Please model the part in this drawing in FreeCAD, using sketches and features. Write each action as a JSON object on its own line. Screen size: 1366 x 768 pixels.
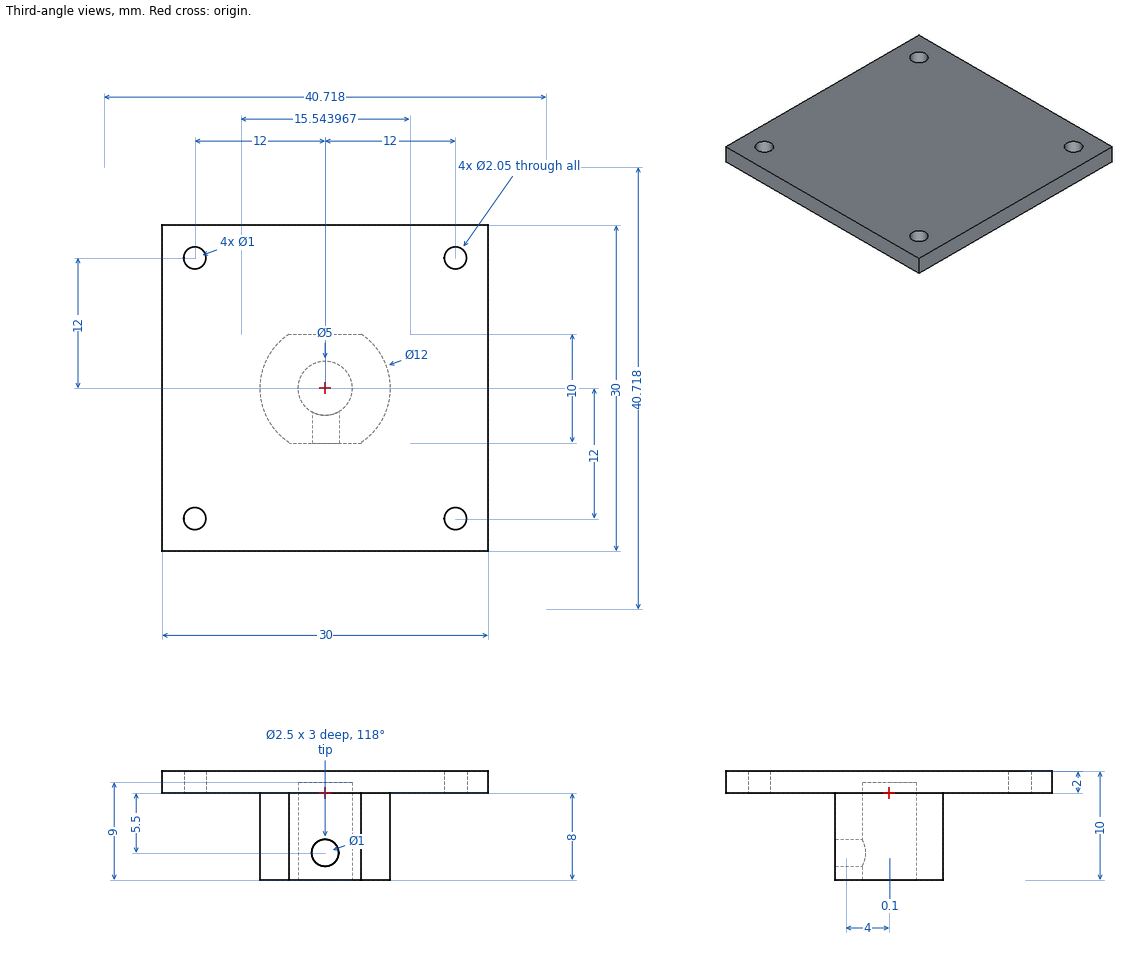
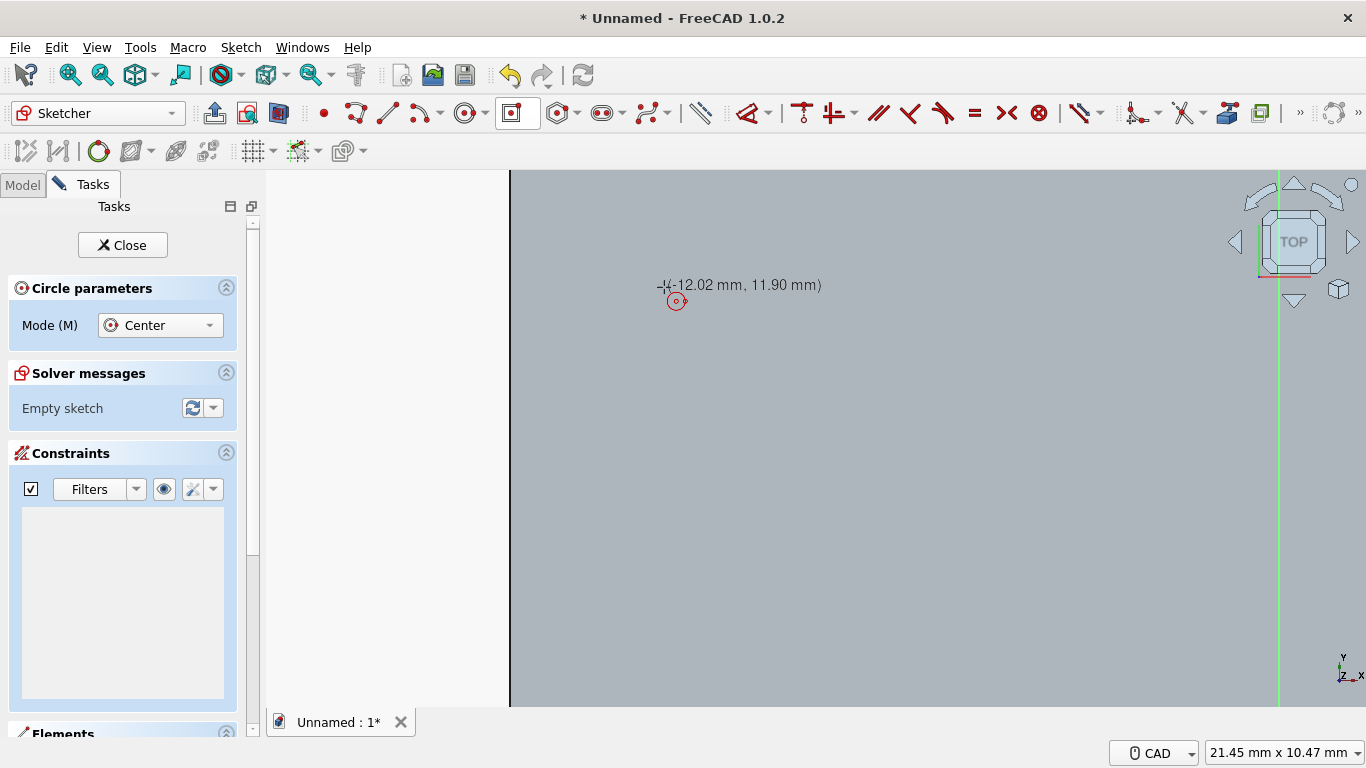
{"action": "scroll", "coordinate": [573, 287], "scroll_direction": "down", "scroll_amount": 7}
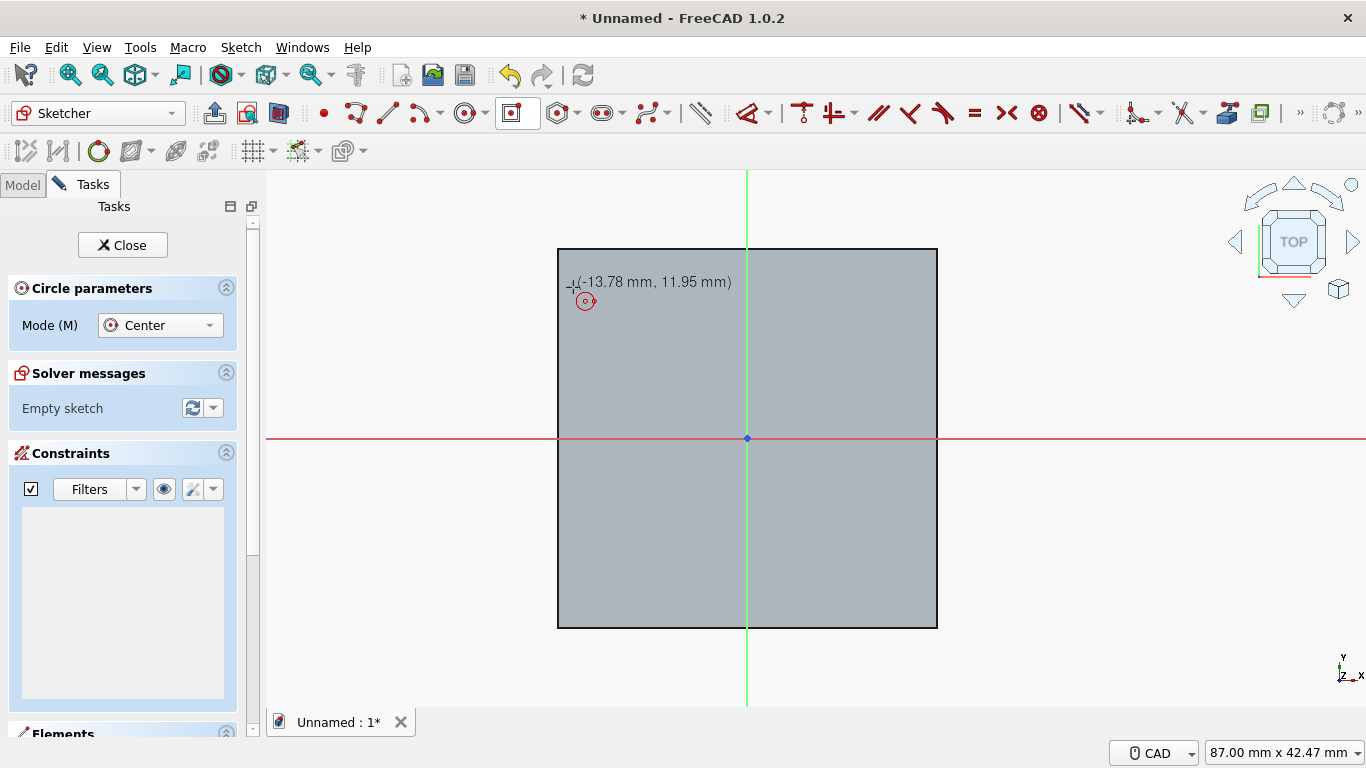
{"action": "left_click", "coordinate": [596, 287]}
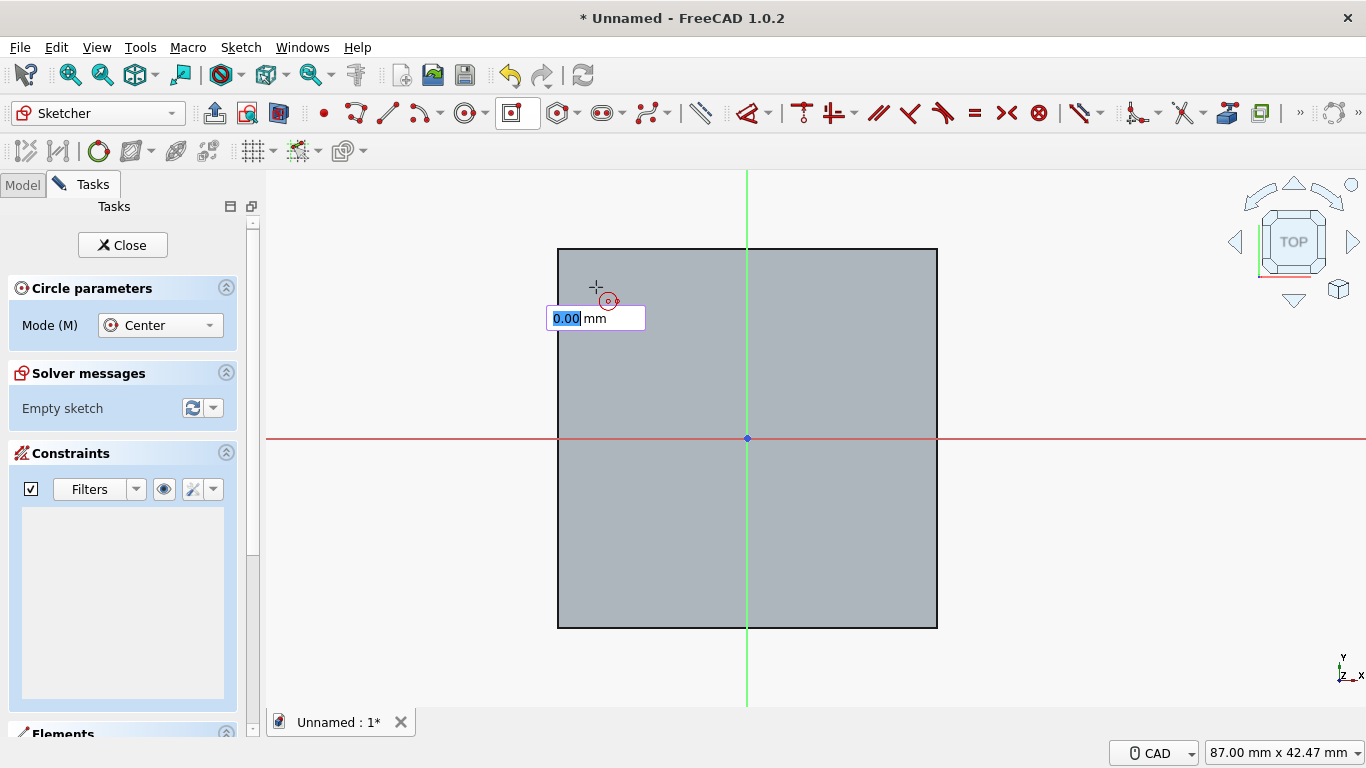
{"action": "scroll", "coordinate": [600, 282], "scroll_direction": "up", "scroll_amount": 5}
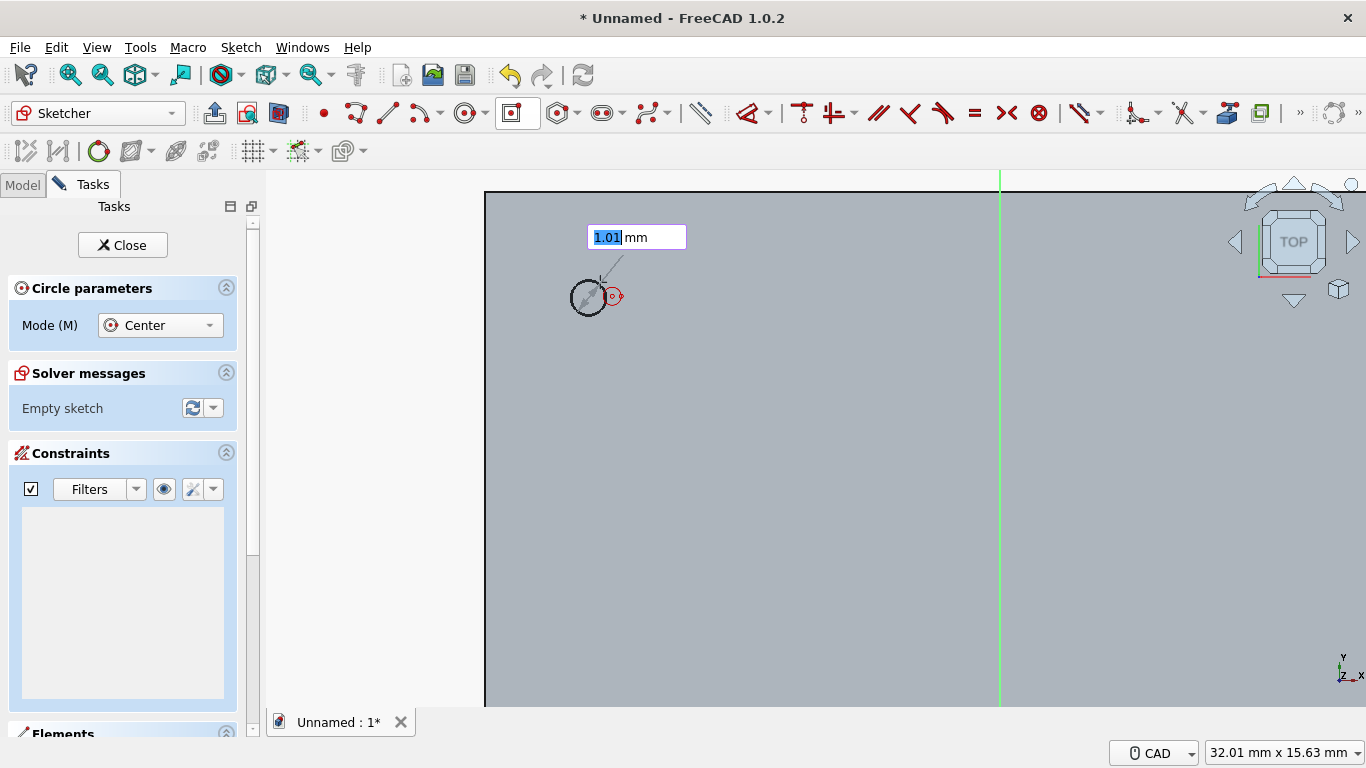
{"action": "left_click", "coordinate": [600, 282]}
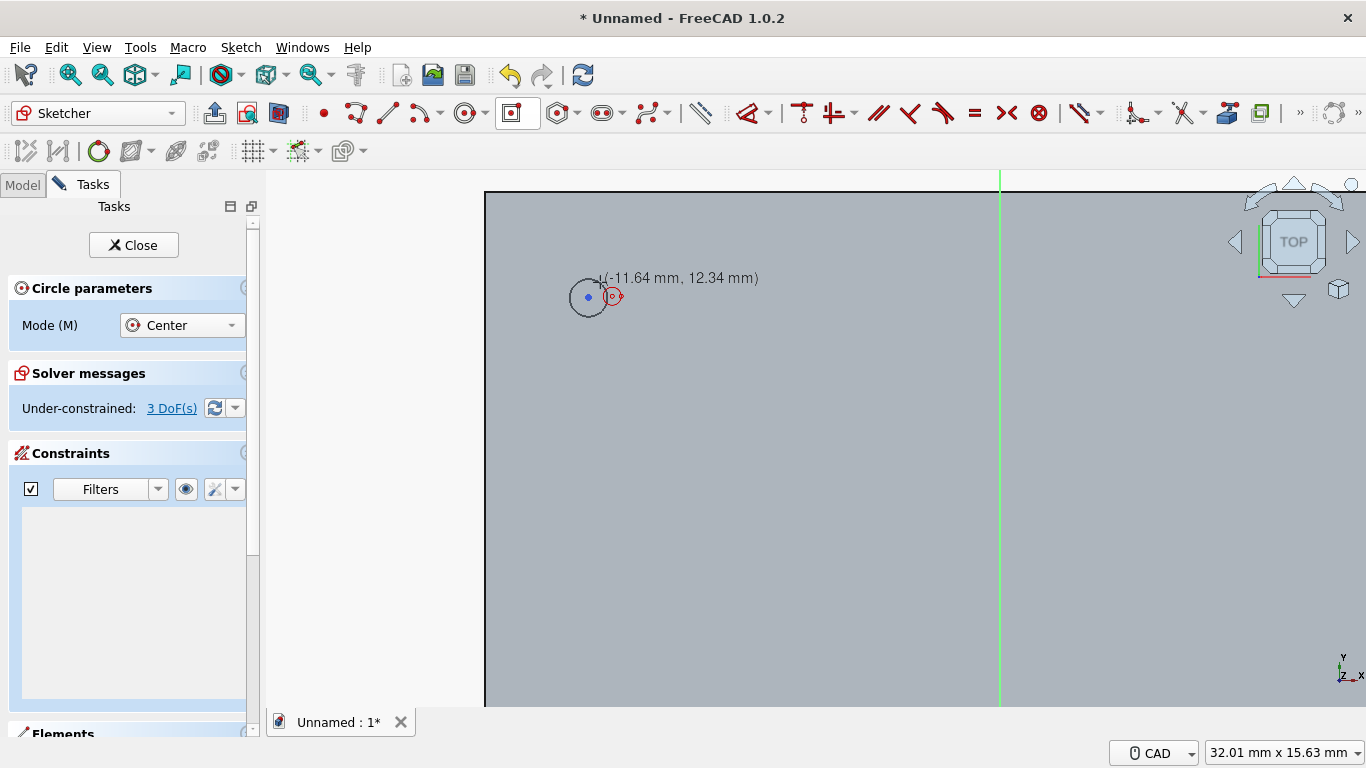
{"action": "scroll", "coordinate": [600, 282], "scroll_direction": "down", "scroll_amount": 5}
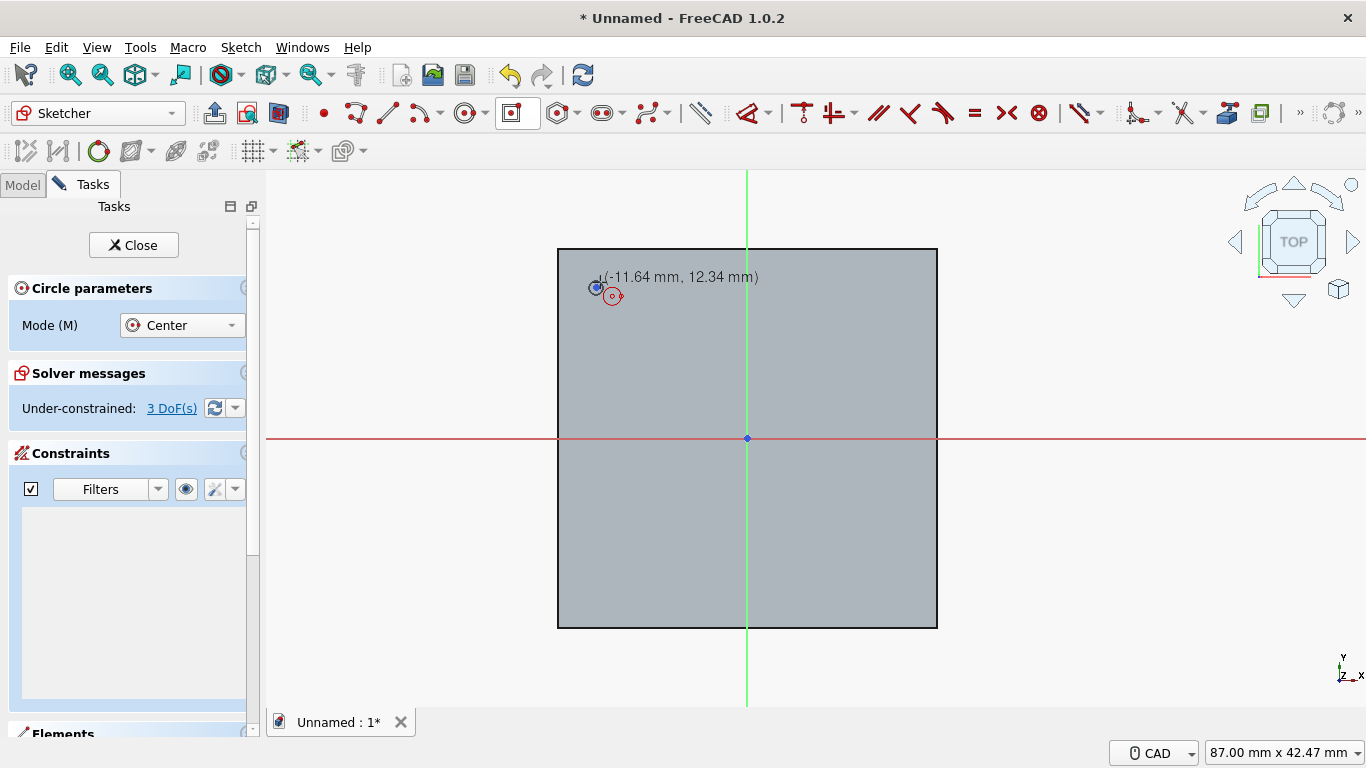
{"action": "scroll", "coordinate": [899, 287], "scroll_direction": "up", "scroll_amount": 7}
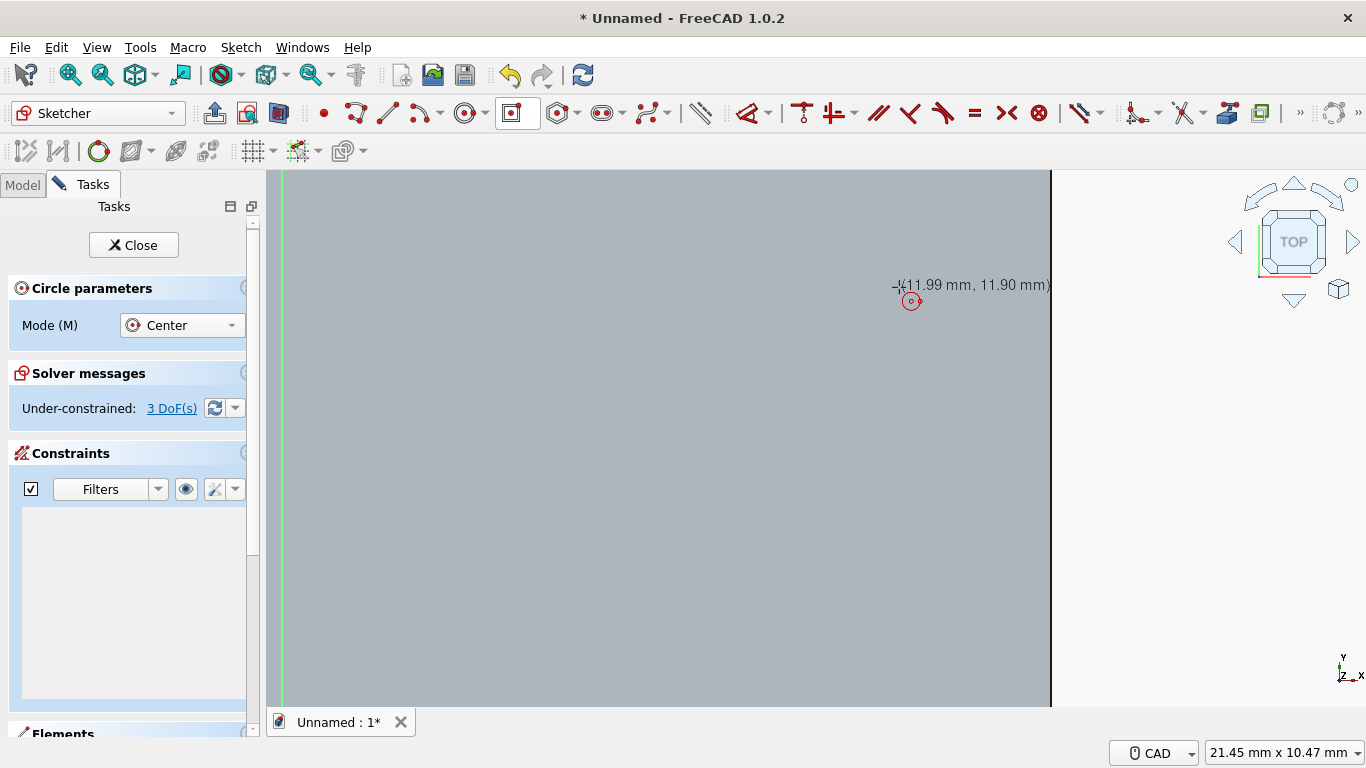
{"action": "scroll", "coordinate": [900, 287], "scroll_direction": "down", "scroll_amount": 7}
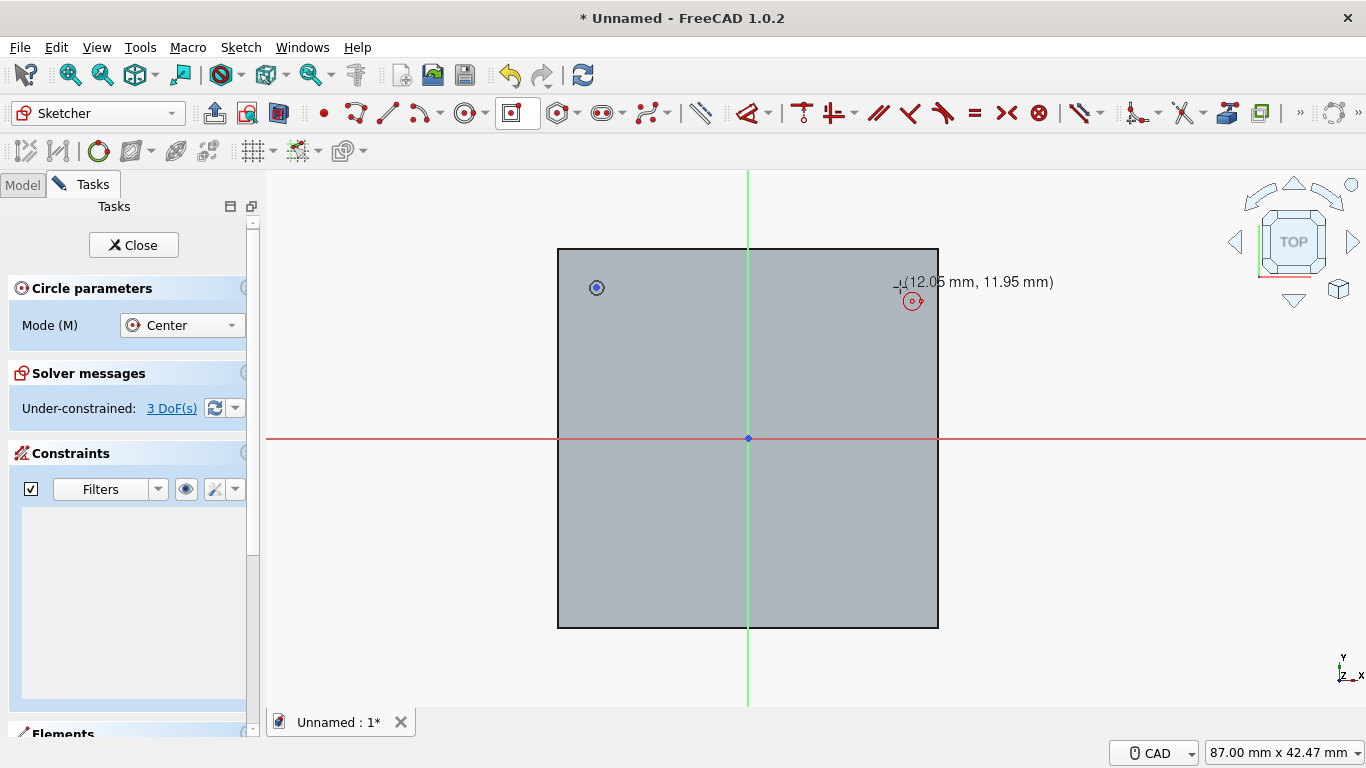
{"action": "left_click", "coordinate": [900, 287]}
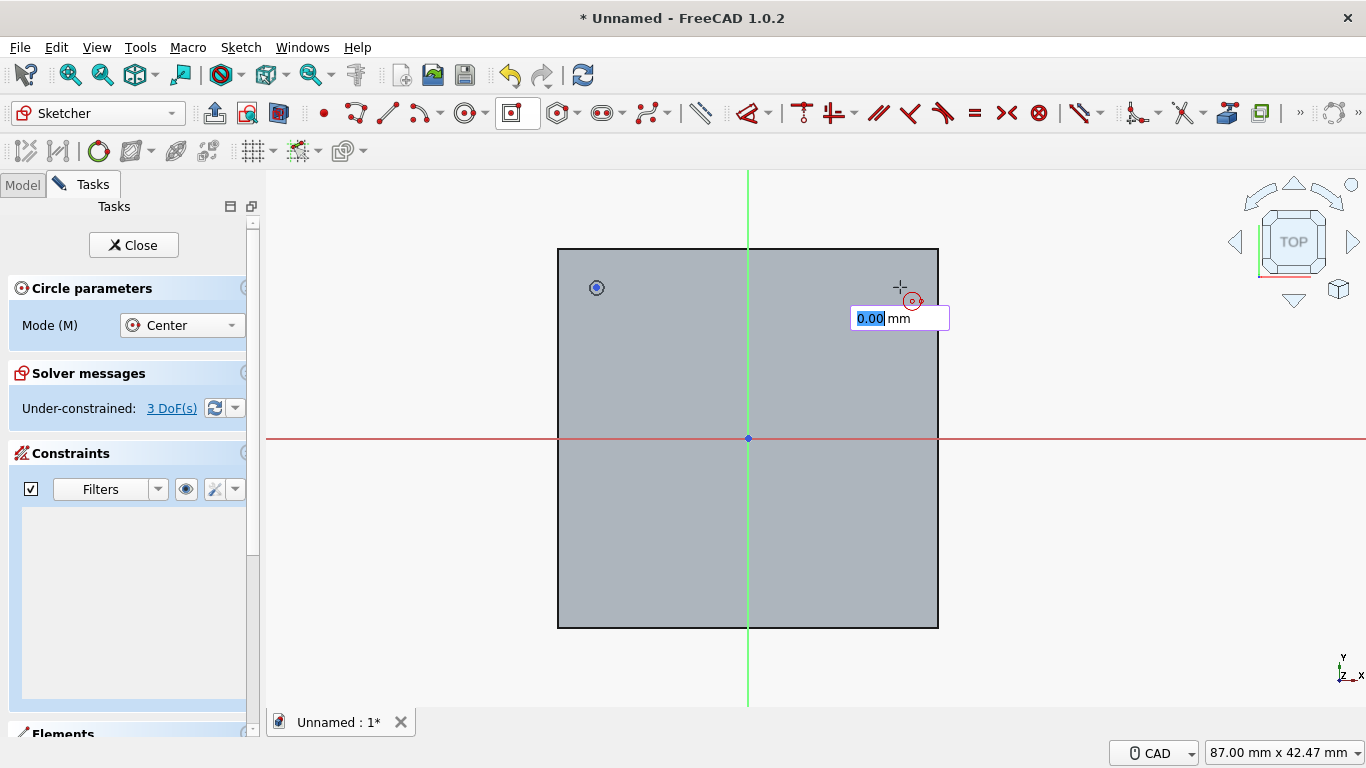
{"action": "scroll", "coordinate": [904, 282], "scroll_direction": "up", "scroll_amount": 5}